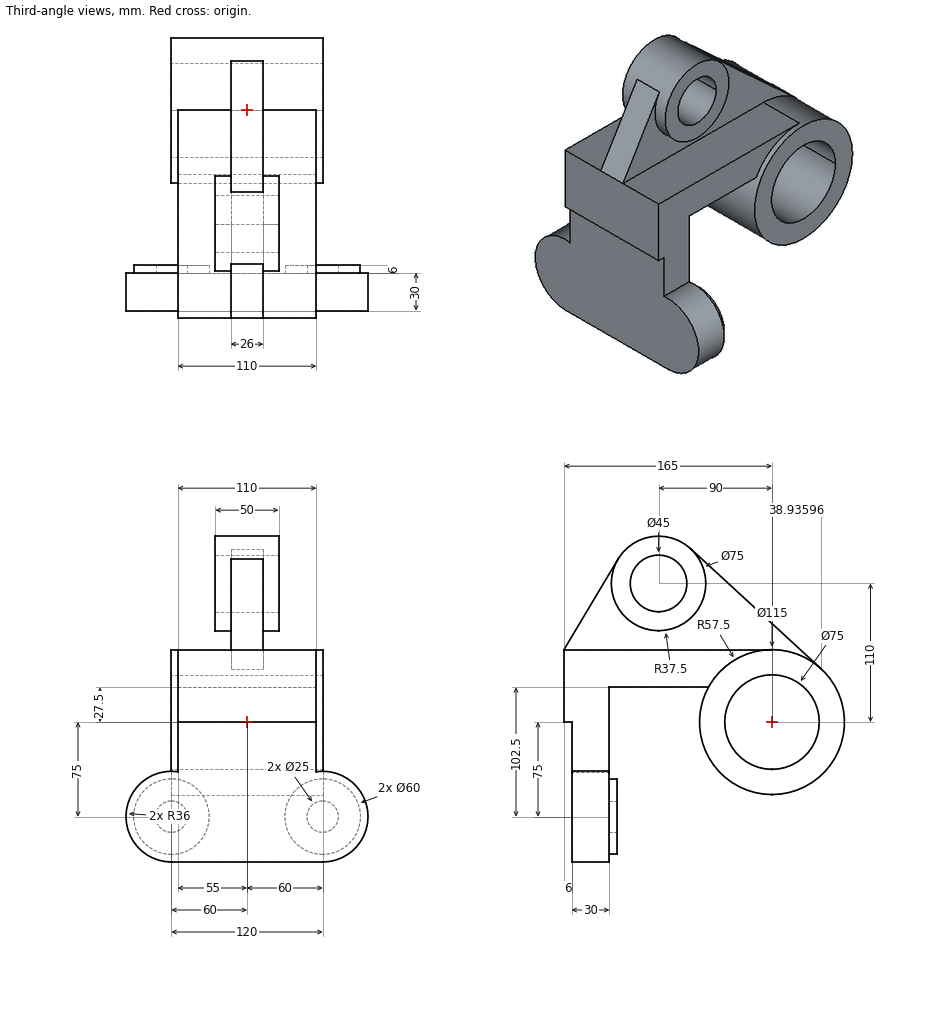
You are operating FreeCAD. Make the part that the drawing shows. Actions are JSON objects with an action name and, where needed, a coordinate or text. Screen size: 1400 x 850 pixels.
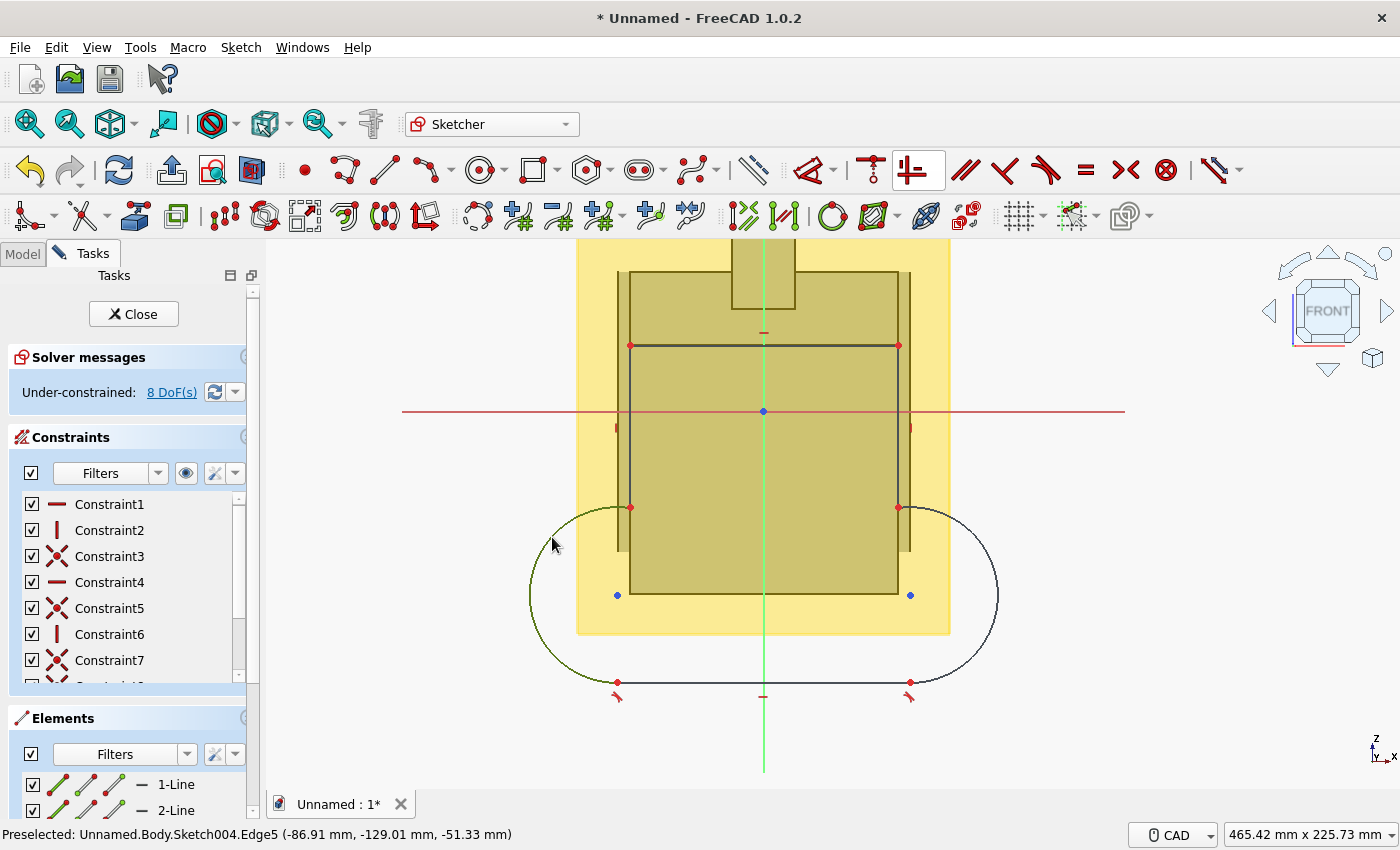
{"action": "left_click", "coordinate": [983, 644]}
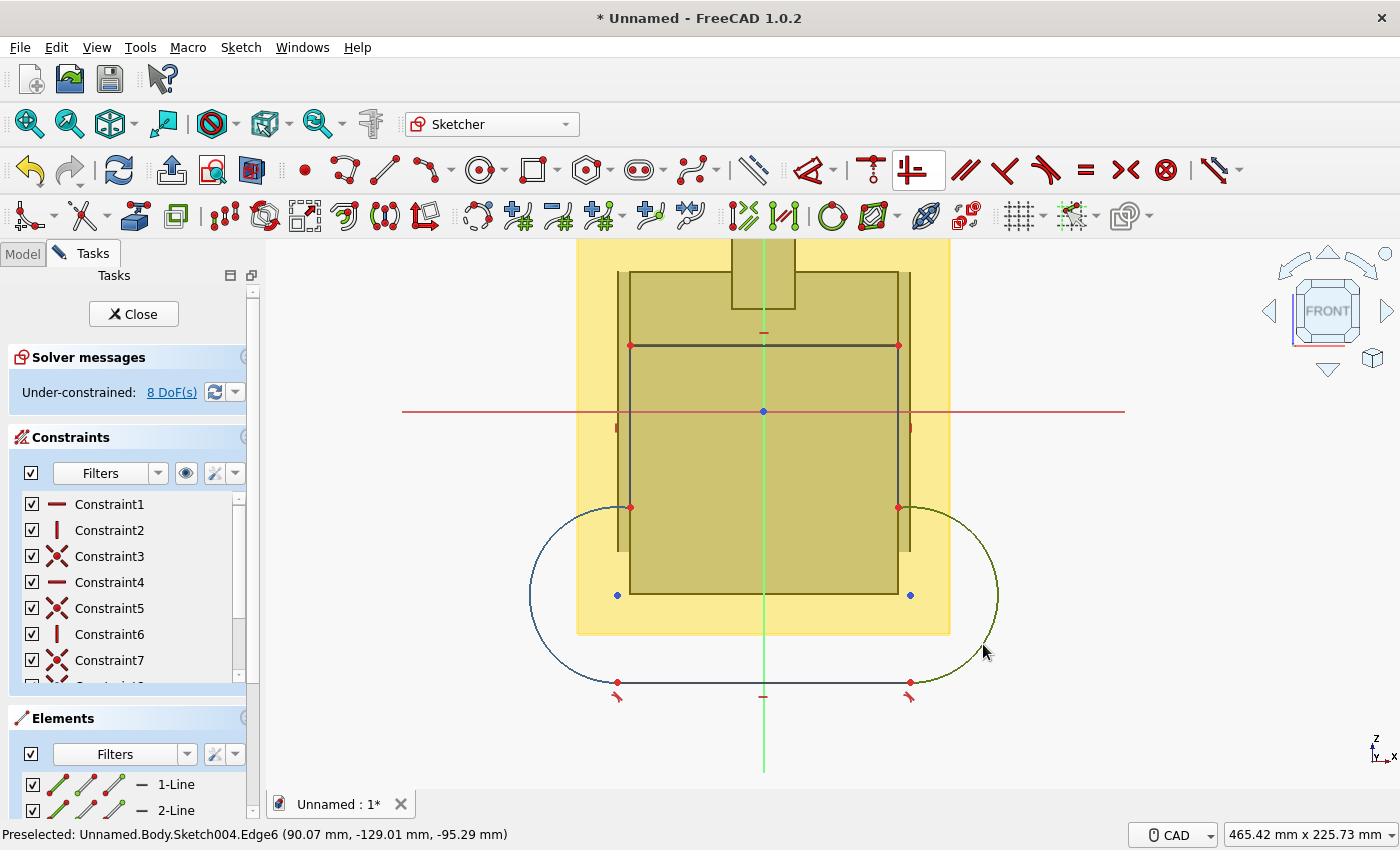
{"action": "key", "text": "e"}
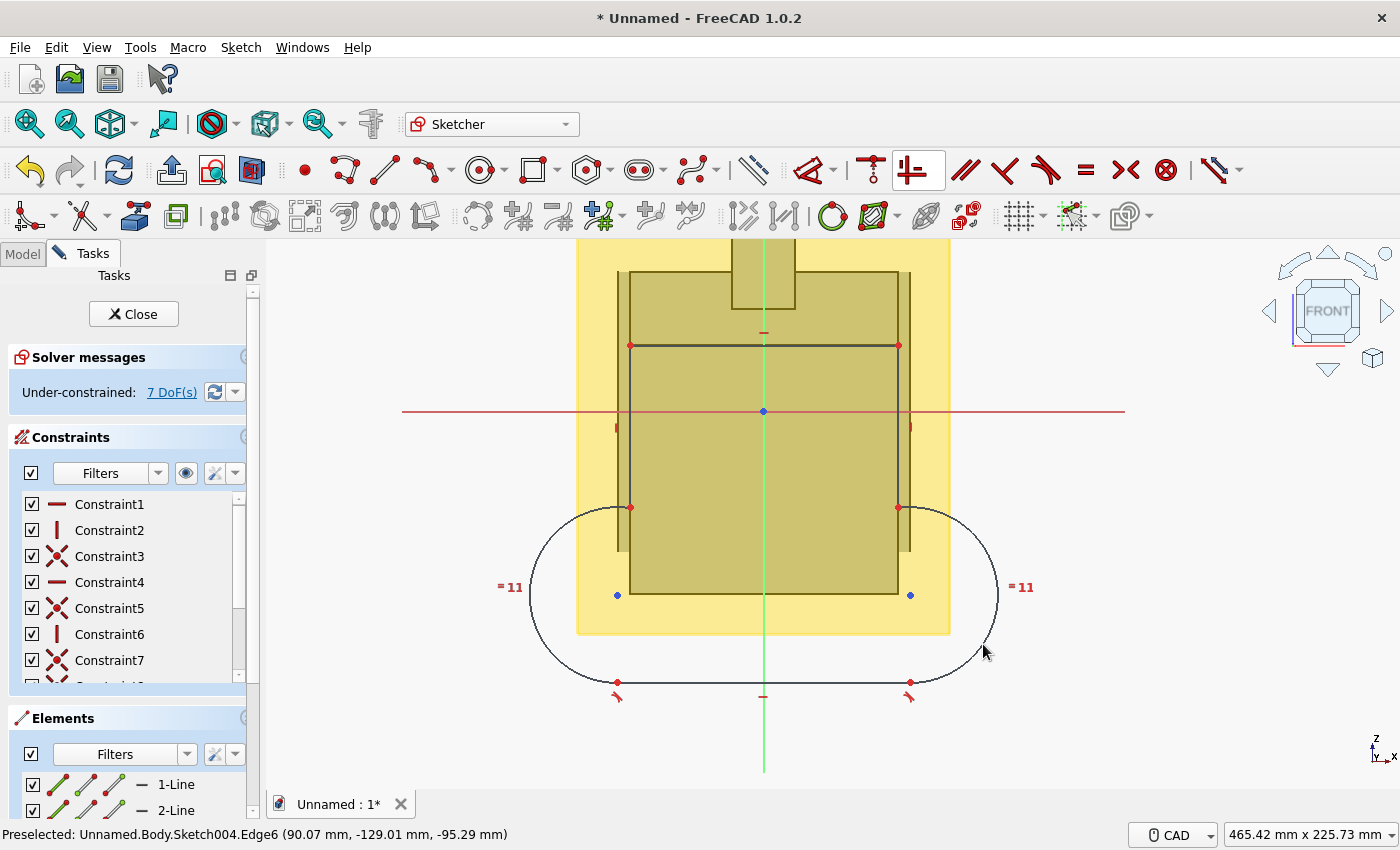
{"action": "left_click", "coordinate": [808, 170]}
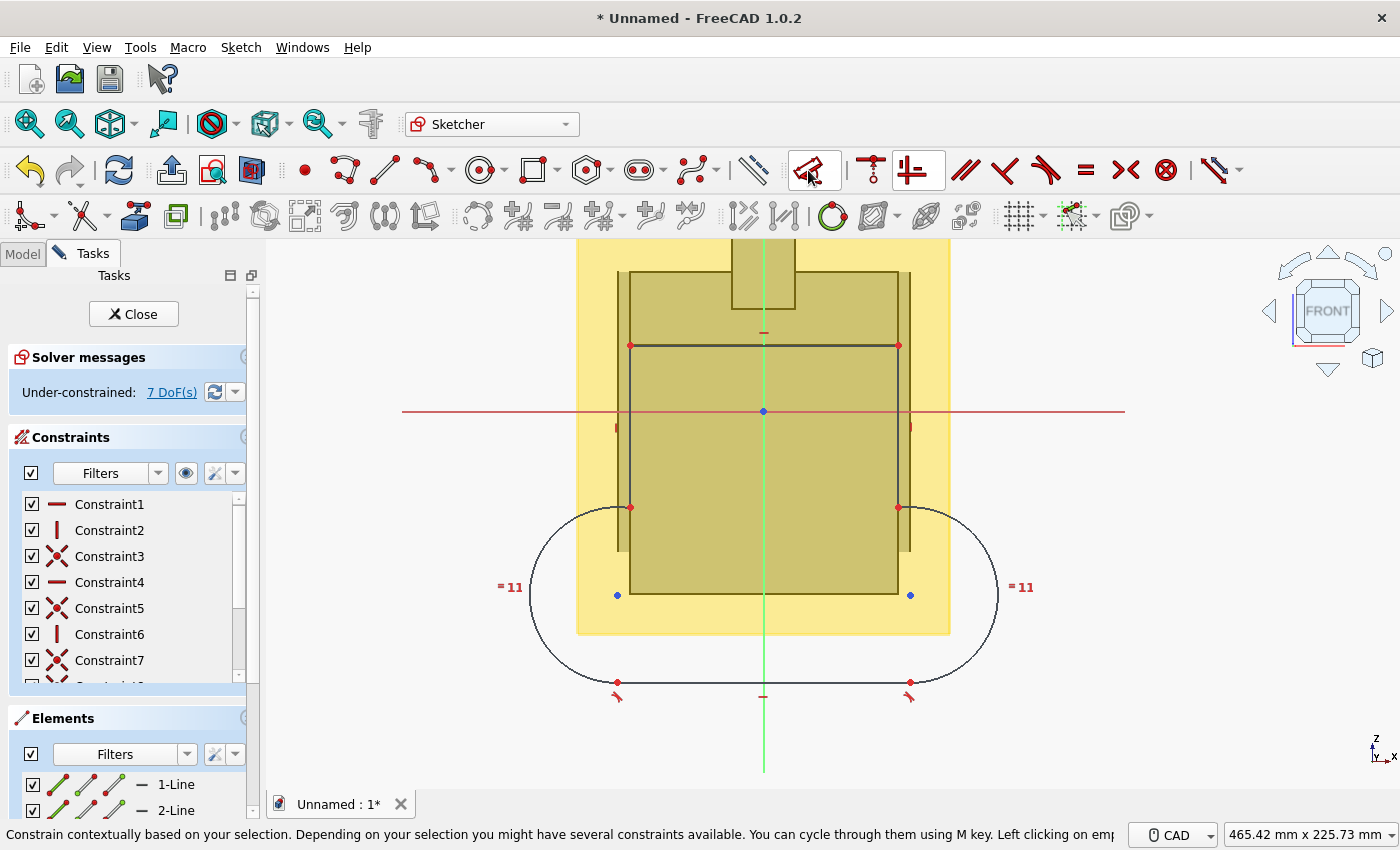
{"action": "left_click", "coordinate": [552, 537]}
{"action": "left_click", "coordinate": [528, 516]}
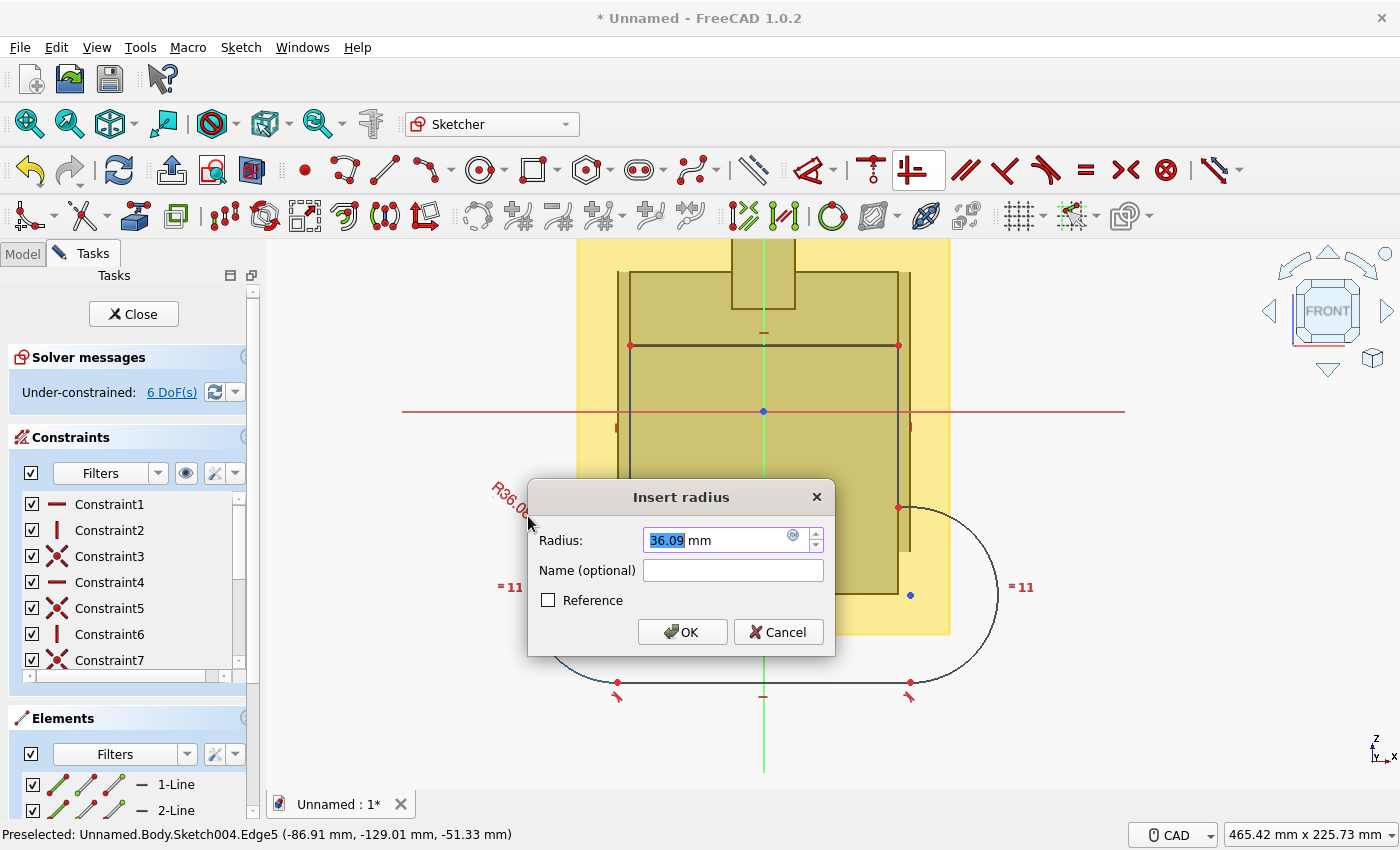
{"action": "type", "text": "36"}
{"action": "key", "text": "Return"}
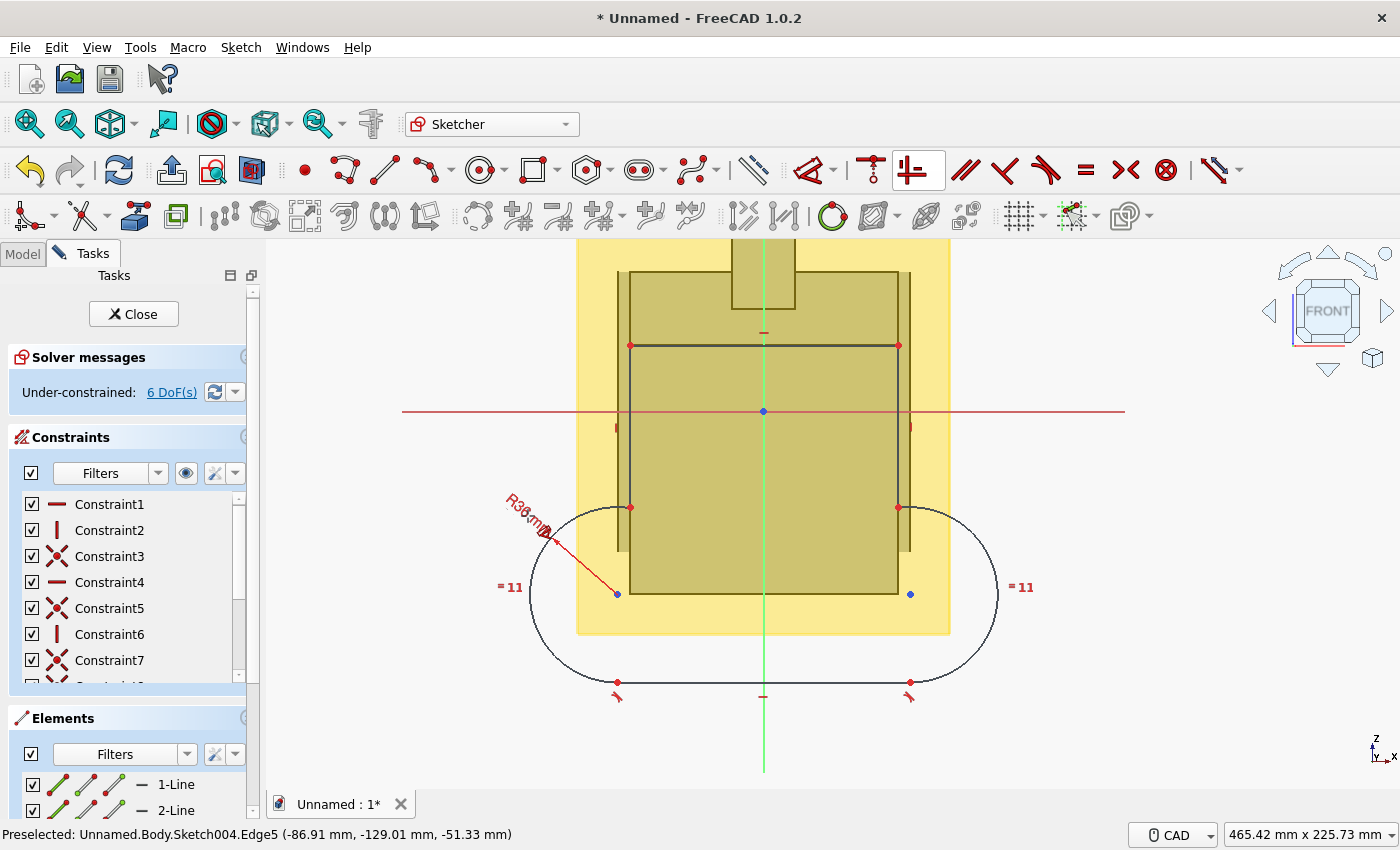
{"action": "left_click", "coordinate": [822, 683]}
{"action": "left_click", "coordinate": [697, 717]}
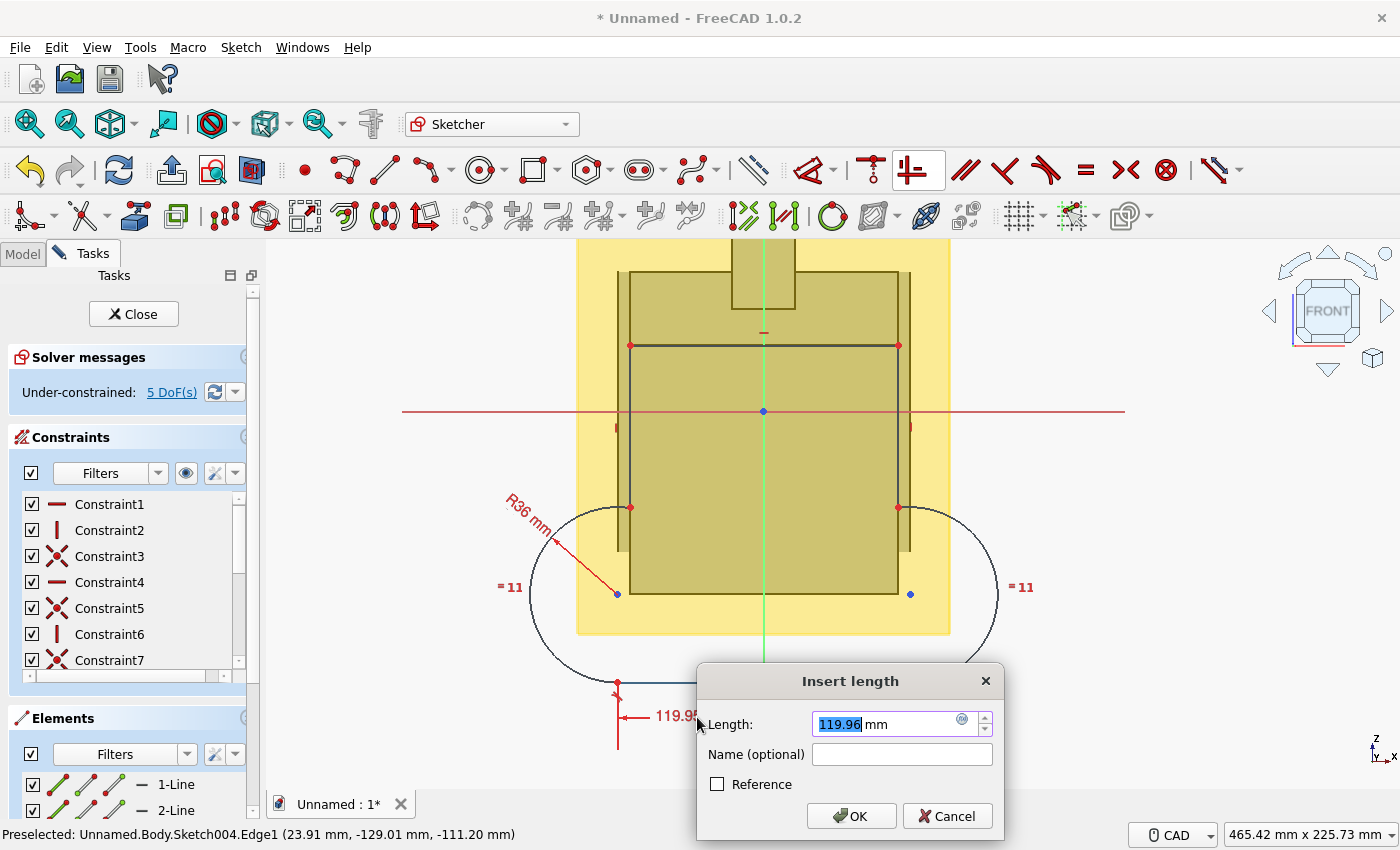
{"action": "type", "text": "120"}
{"action": "key", "text": "Return"}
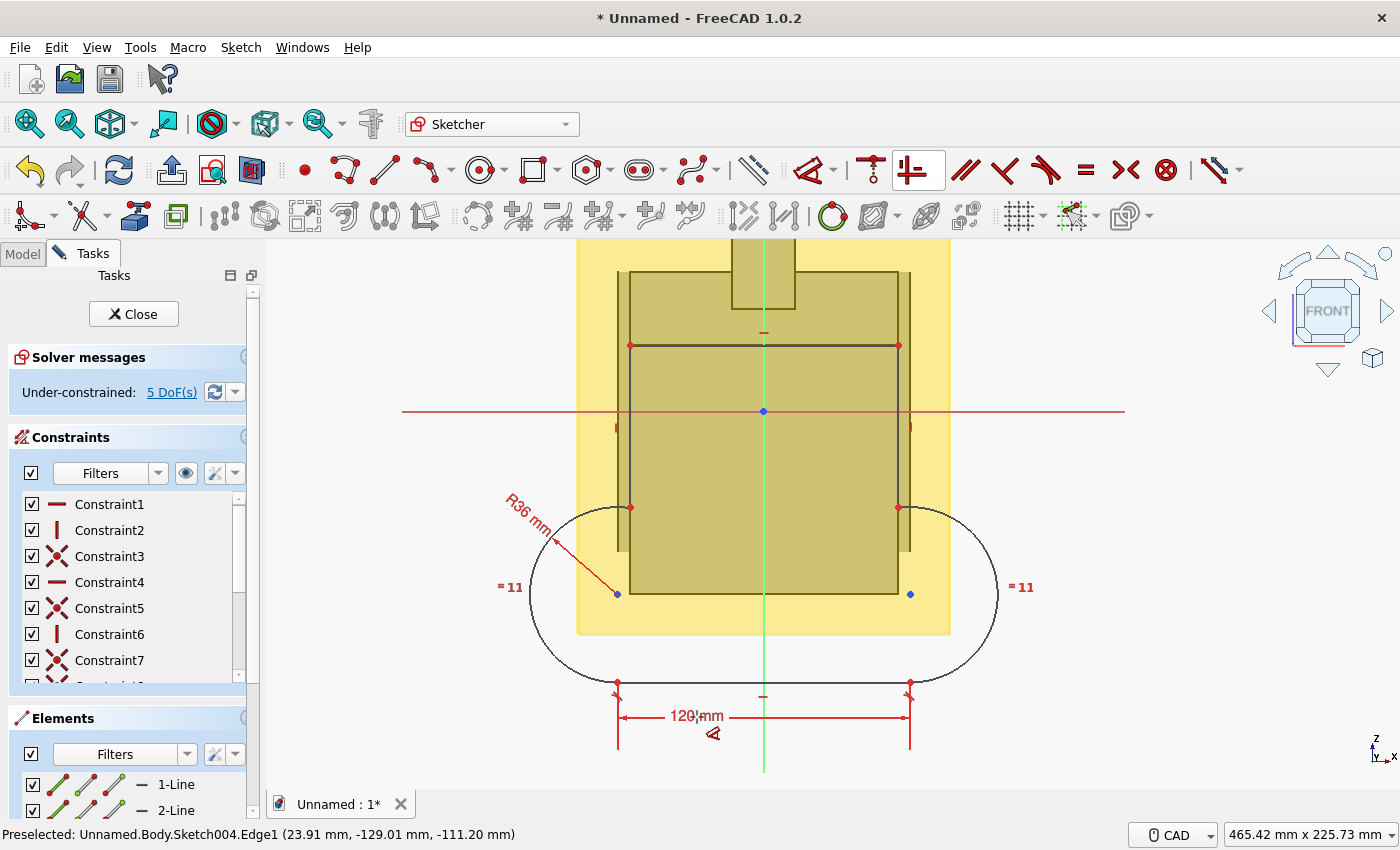
{"action": "left_click", "coordinate": [710, 346]}
{"action": "left_click", "coordinate": [702, 312]}